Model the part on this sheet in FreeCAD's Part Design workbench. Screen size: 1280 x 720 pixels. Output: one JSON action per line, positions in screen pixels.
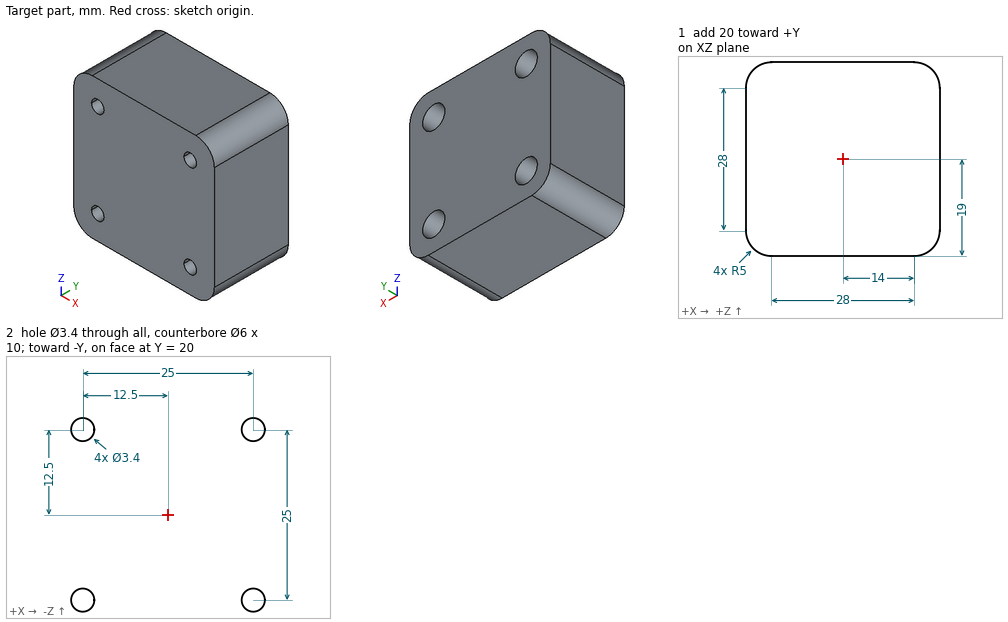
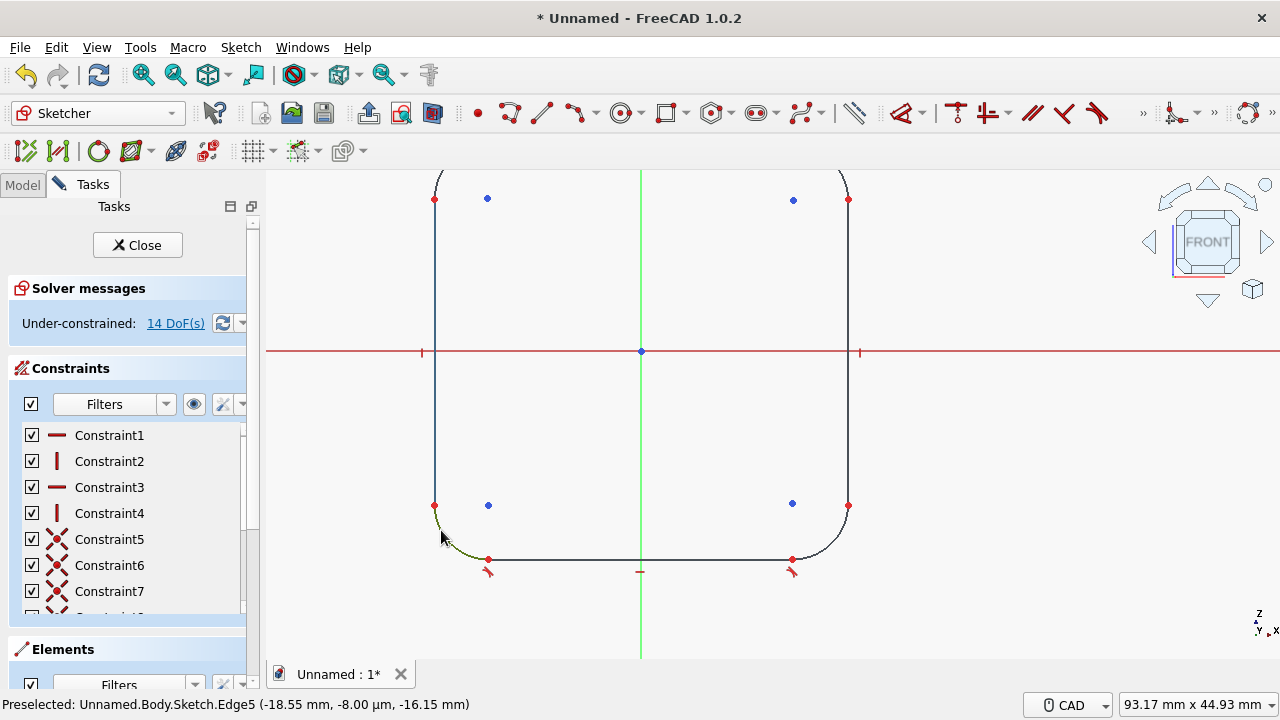
{"action": "left_click", "coordinate": [1098, 114]}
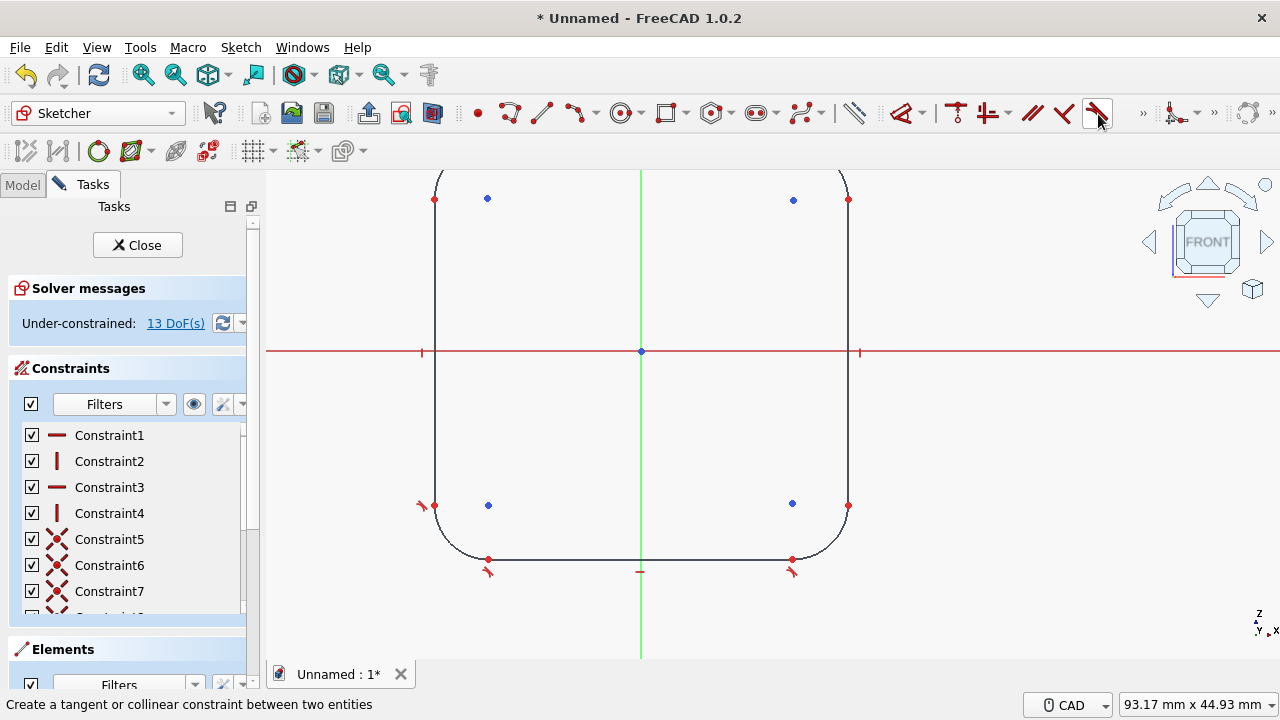
{"action": "left_click", "coordinate": [435, 414]}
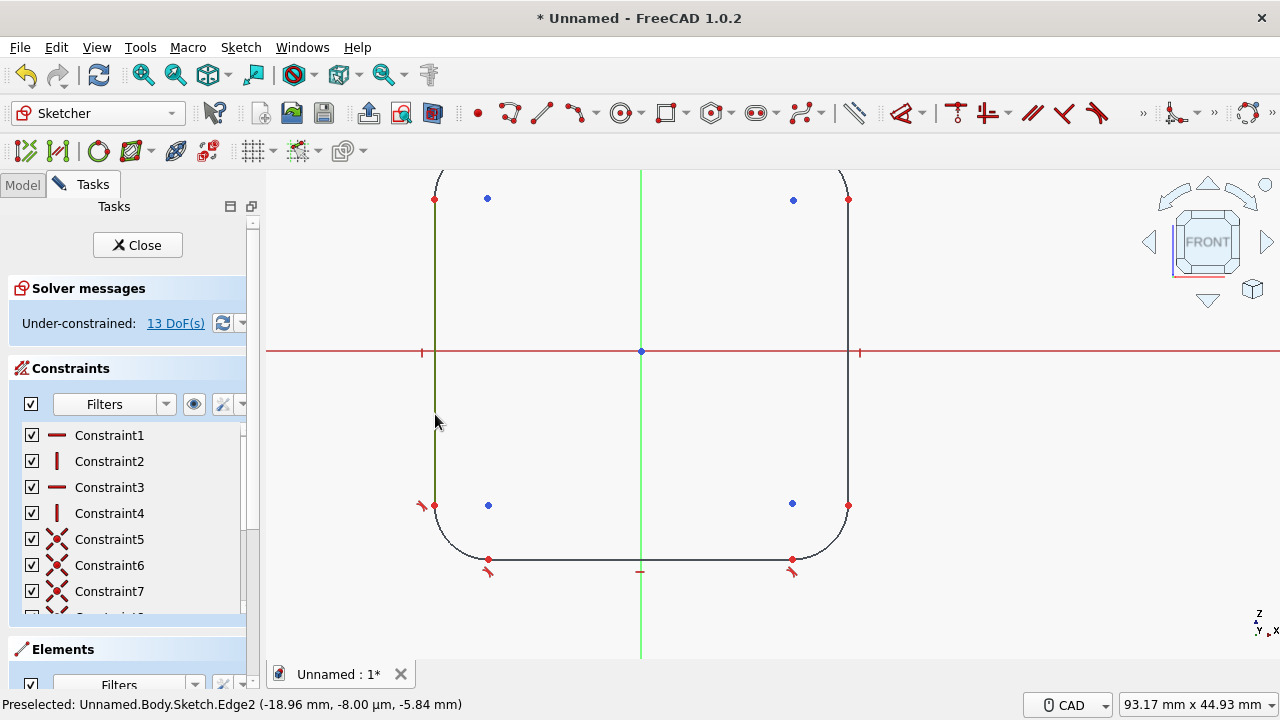
{"action": "scroll", "coordinate": [833, 543], "scroll_direction": "down", "scroll_amount": 2}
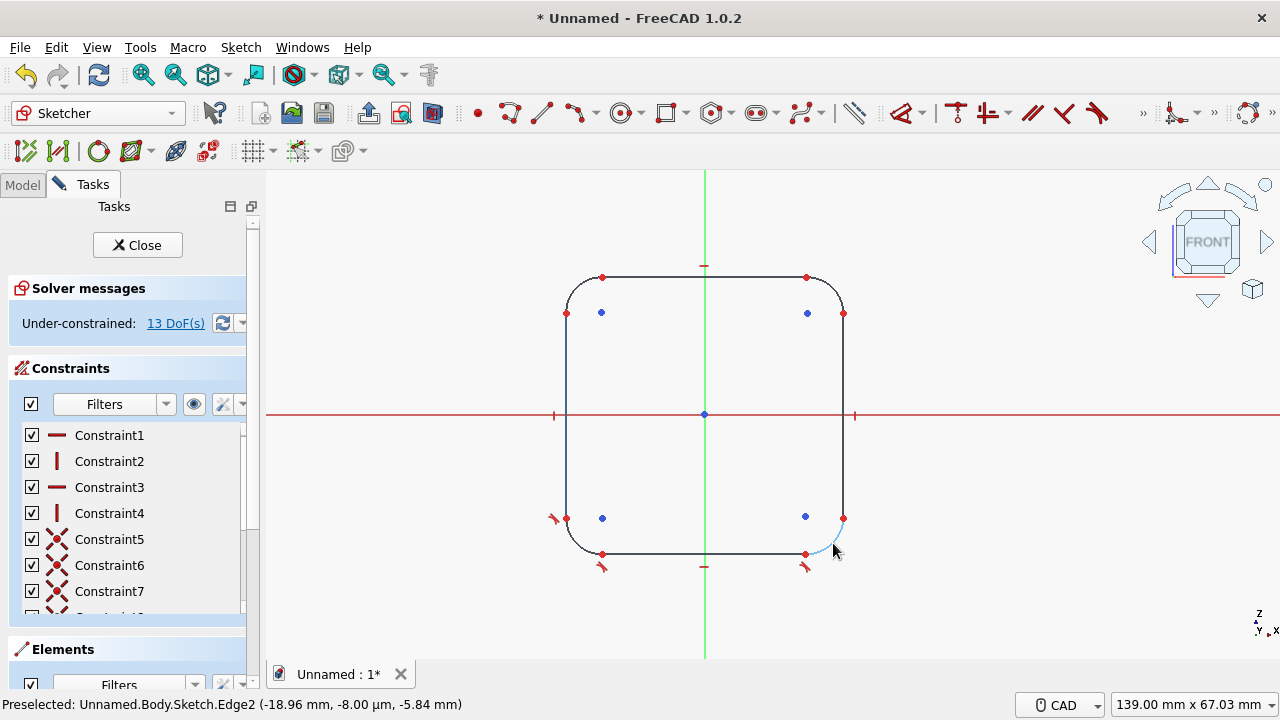
{"action": "left_click", "coordinate": [586, 281]}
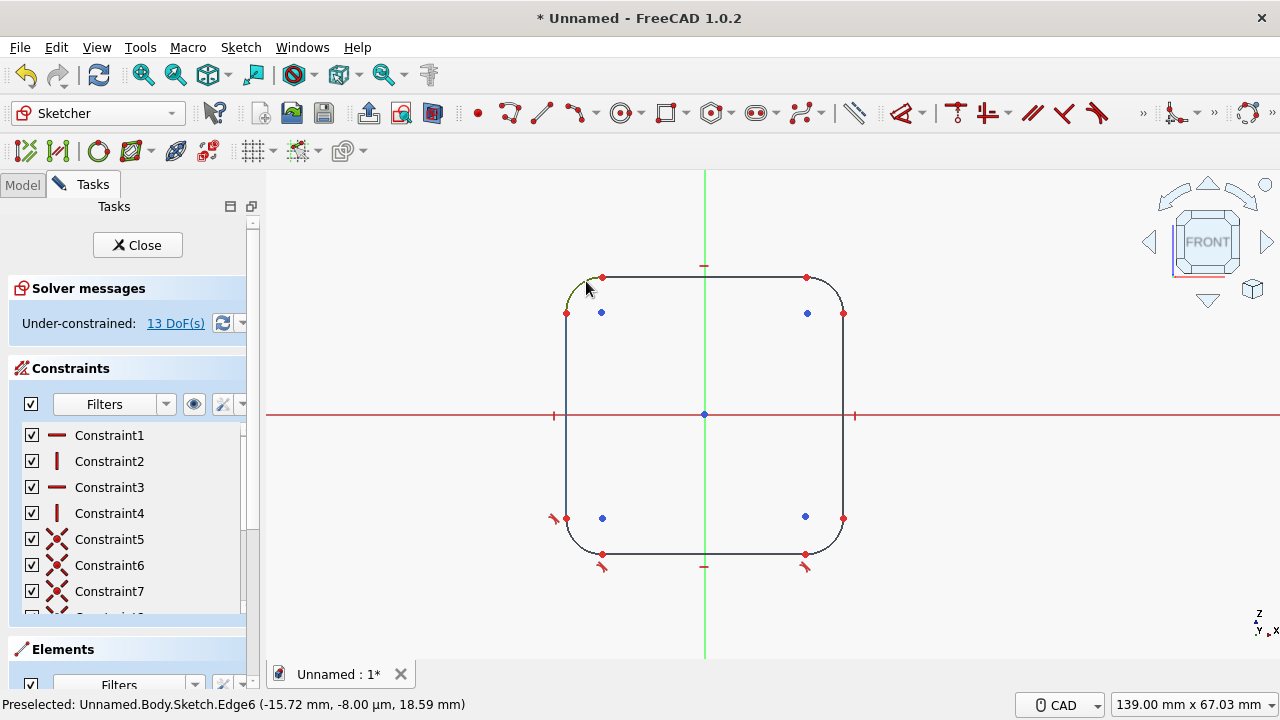
{"action": "left_click", "coordinate": [1098, 114]}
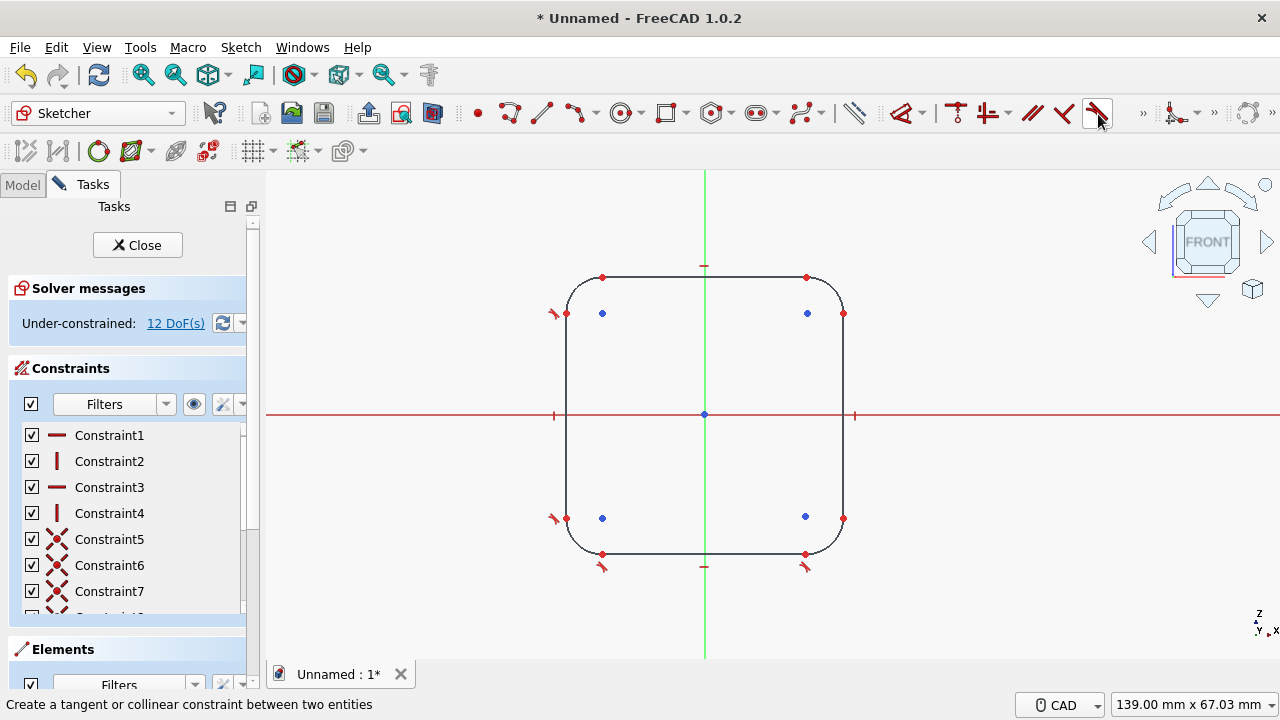
{"action": "left_click", "coordinate": [664, 277]}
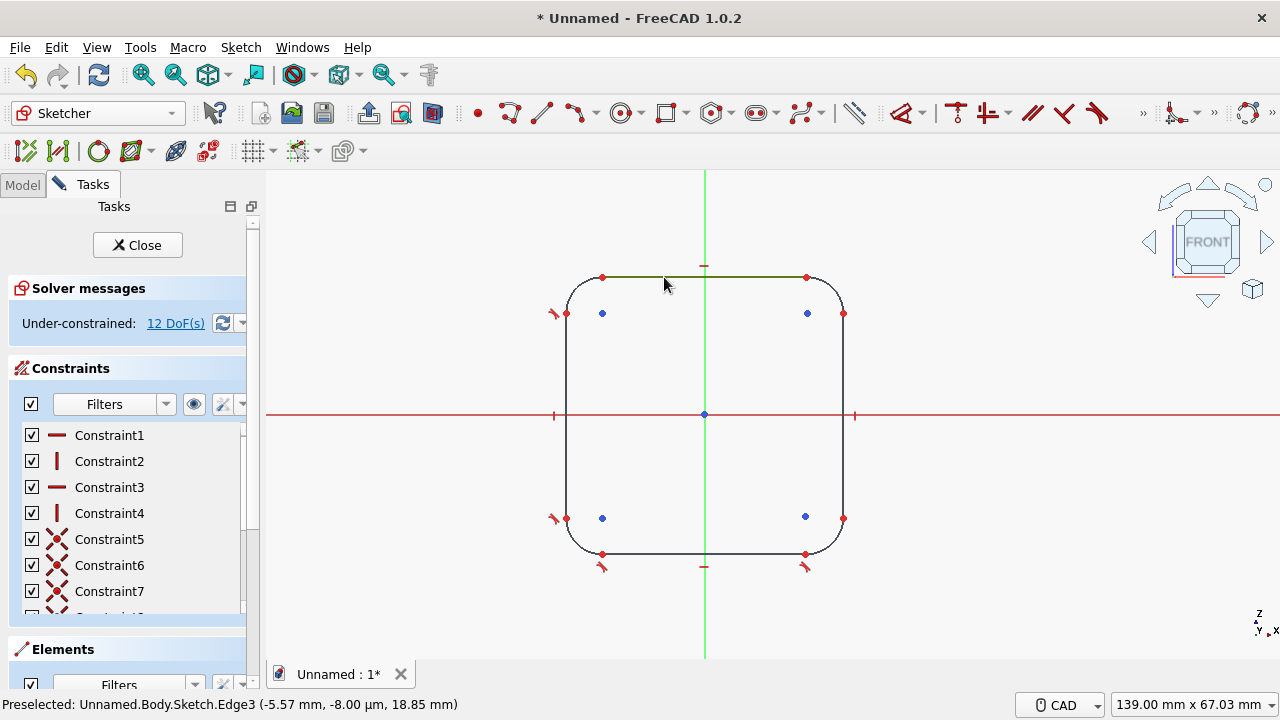
{"action": "left_click", "coordinate": [586, 281]}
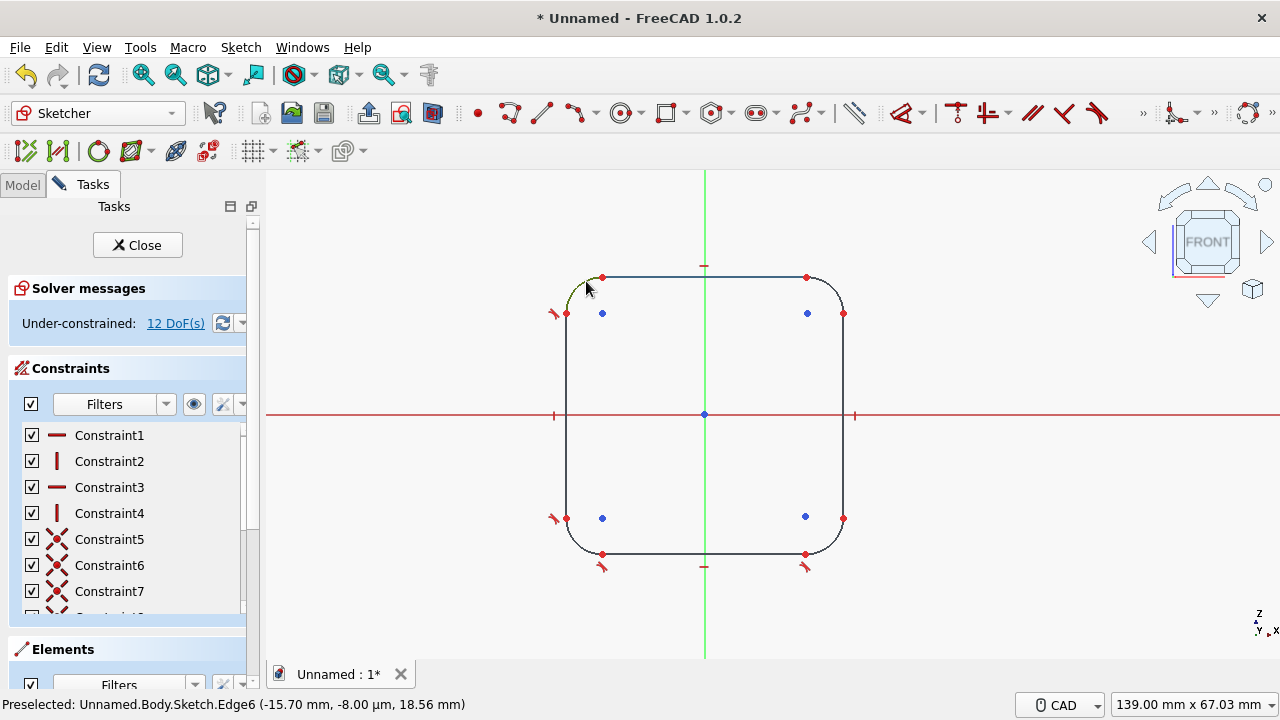
{"action": "left_click", "coordinate": [1098, 114]}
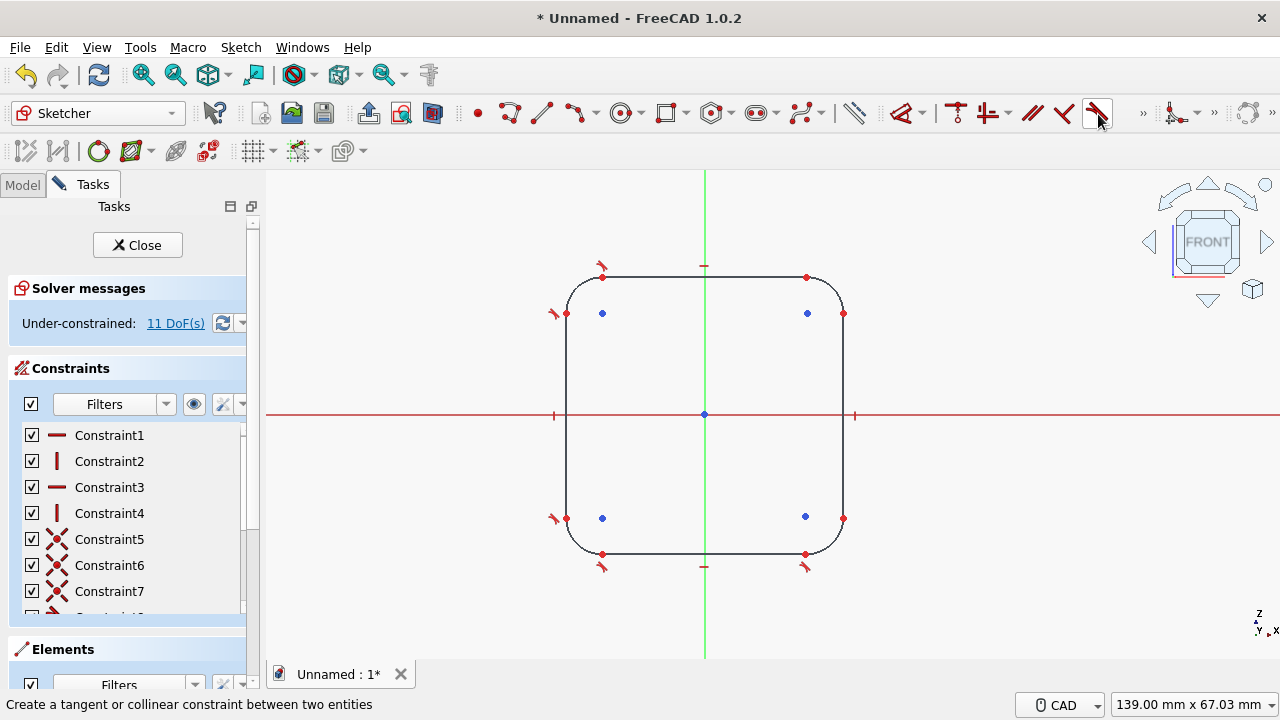
{"action": "left_click", "coordinate": [664, 277]}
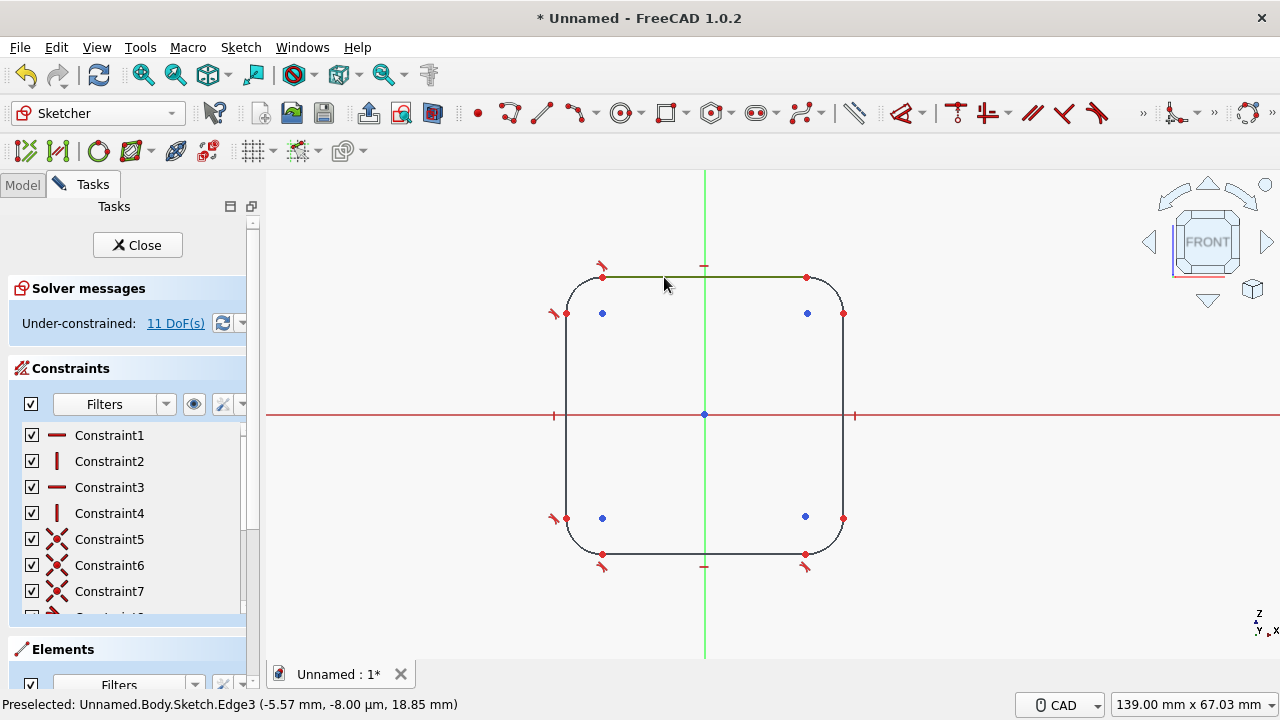
{"action": "left_click", "coordinate": [839, 297]}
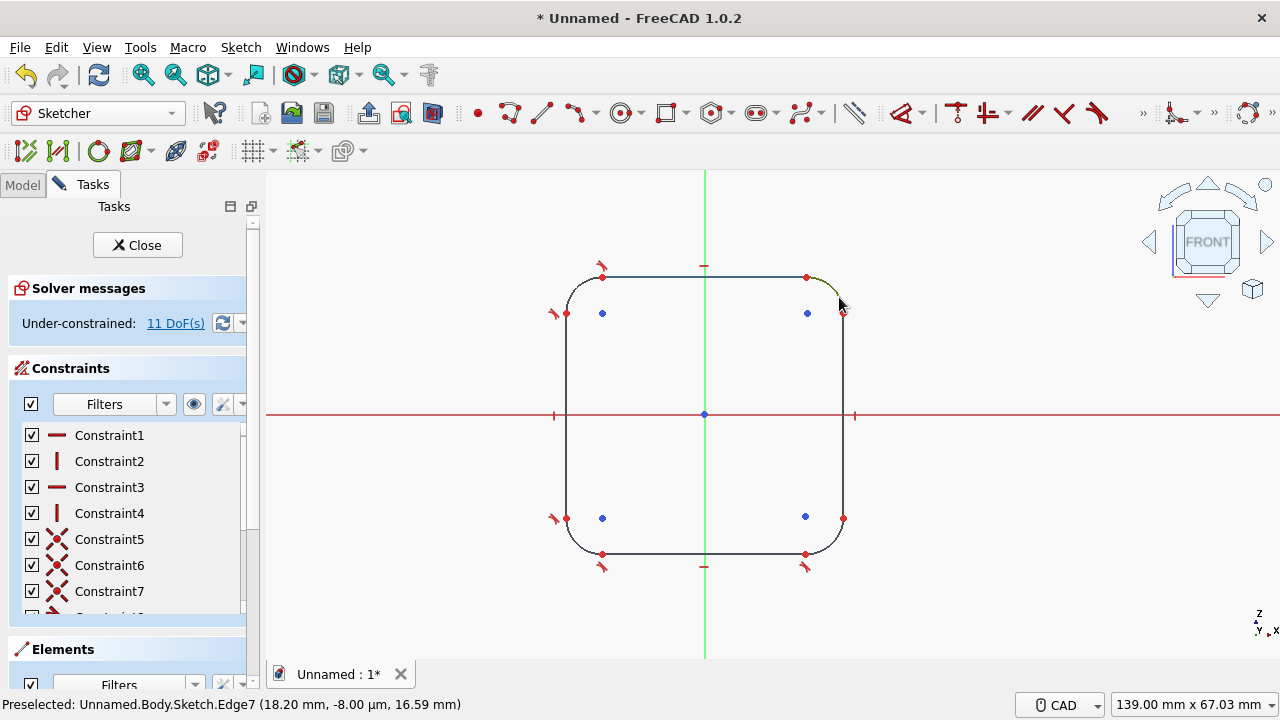
{"action": "left_click", "coordinate": [1098, 114]}